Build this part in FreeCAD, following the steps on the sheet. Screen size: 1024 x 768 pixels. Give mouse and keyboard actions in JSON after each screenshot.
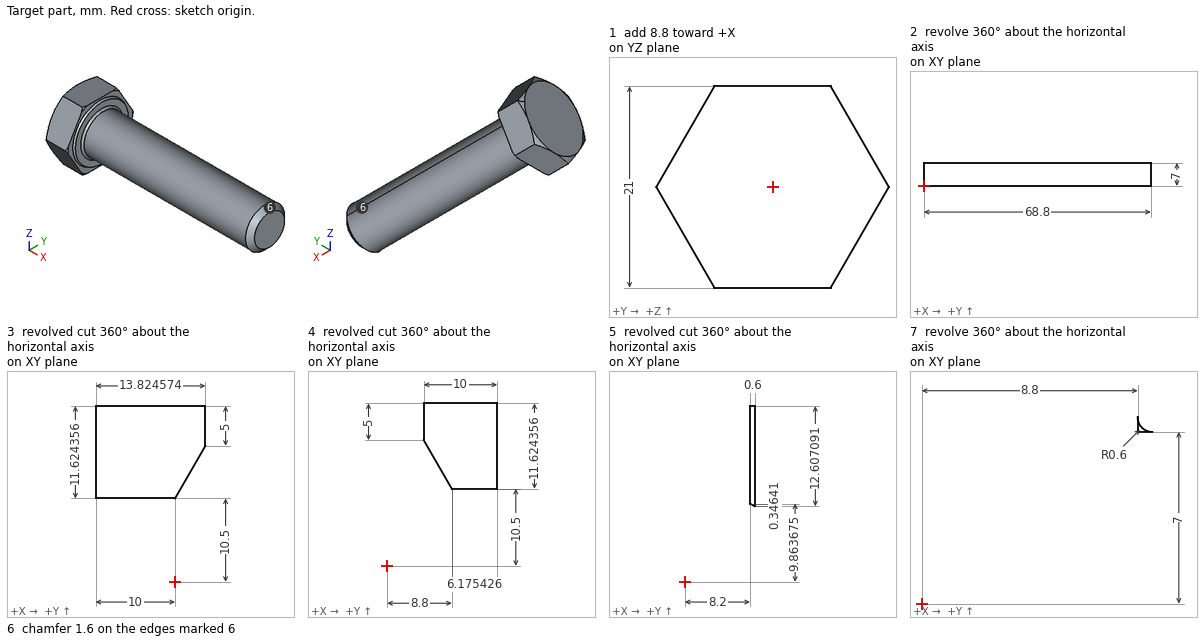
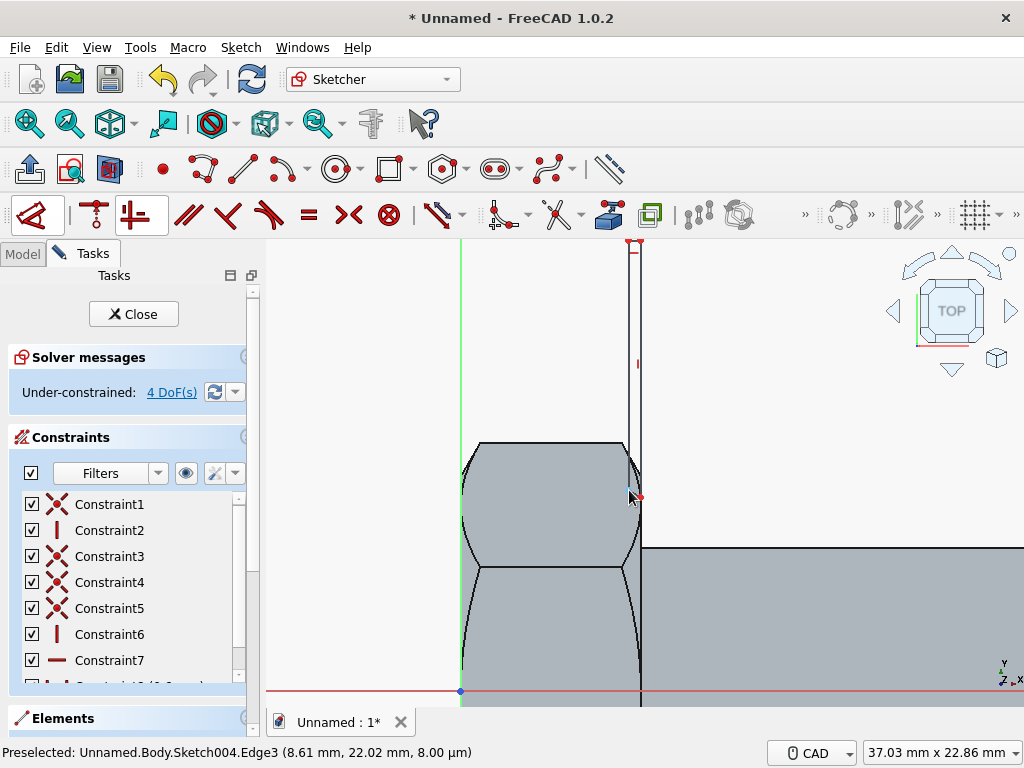
{"action": "left_click", "coordinate": [629, 490]}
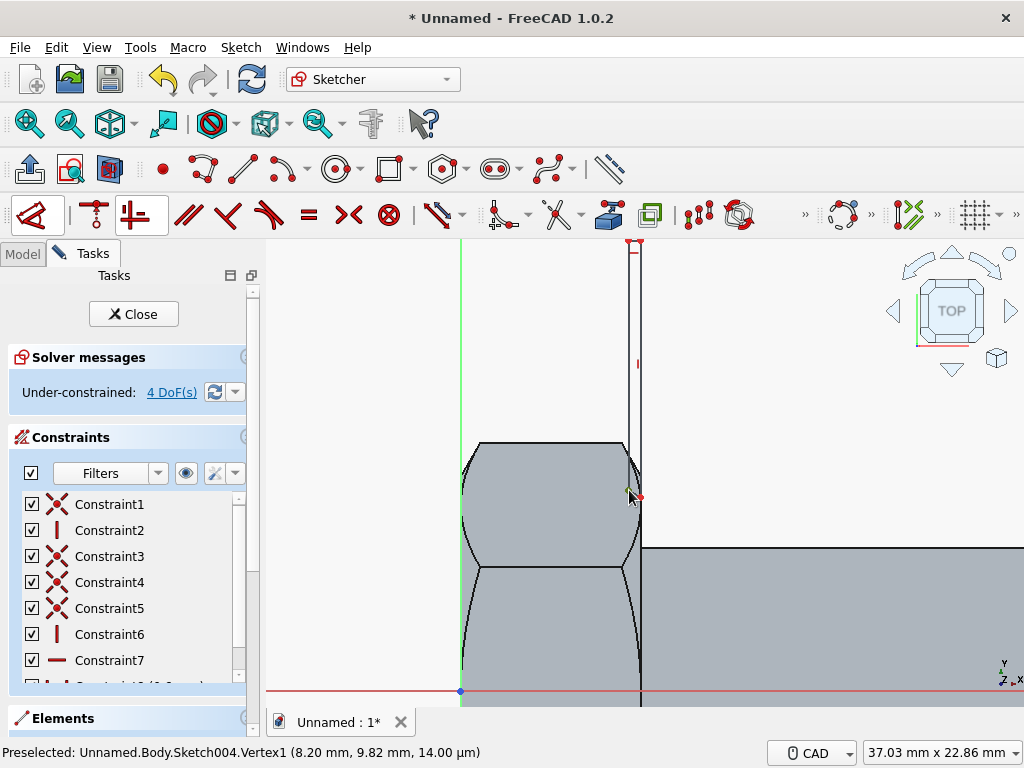
{"action": "left_click", "coordinate": [58, 216]}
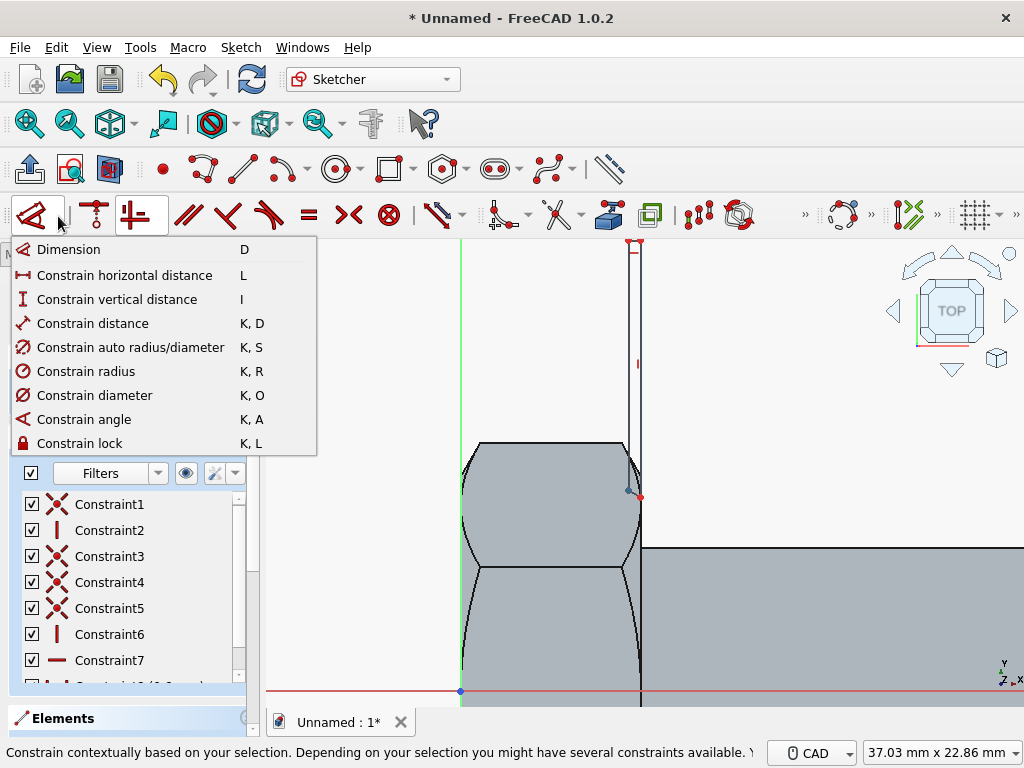
{"action": "left_click", "coordinate": [164, 275]}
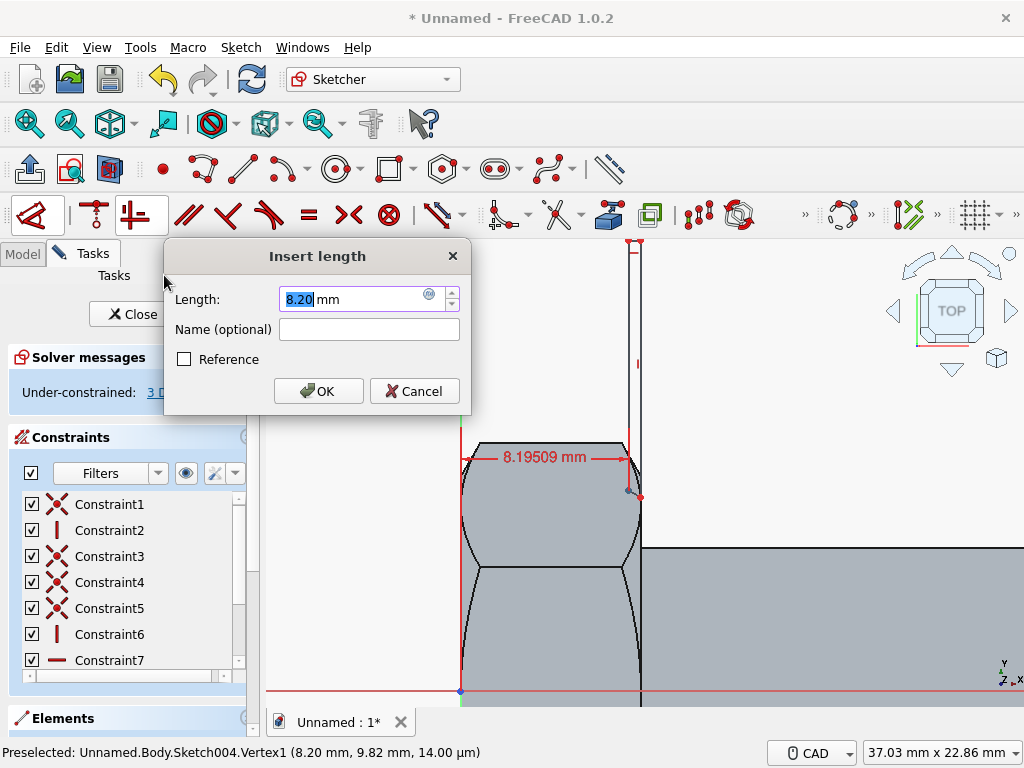
{"action": "type", "text": "8.2"}
{"action": "key", "text": "Return"}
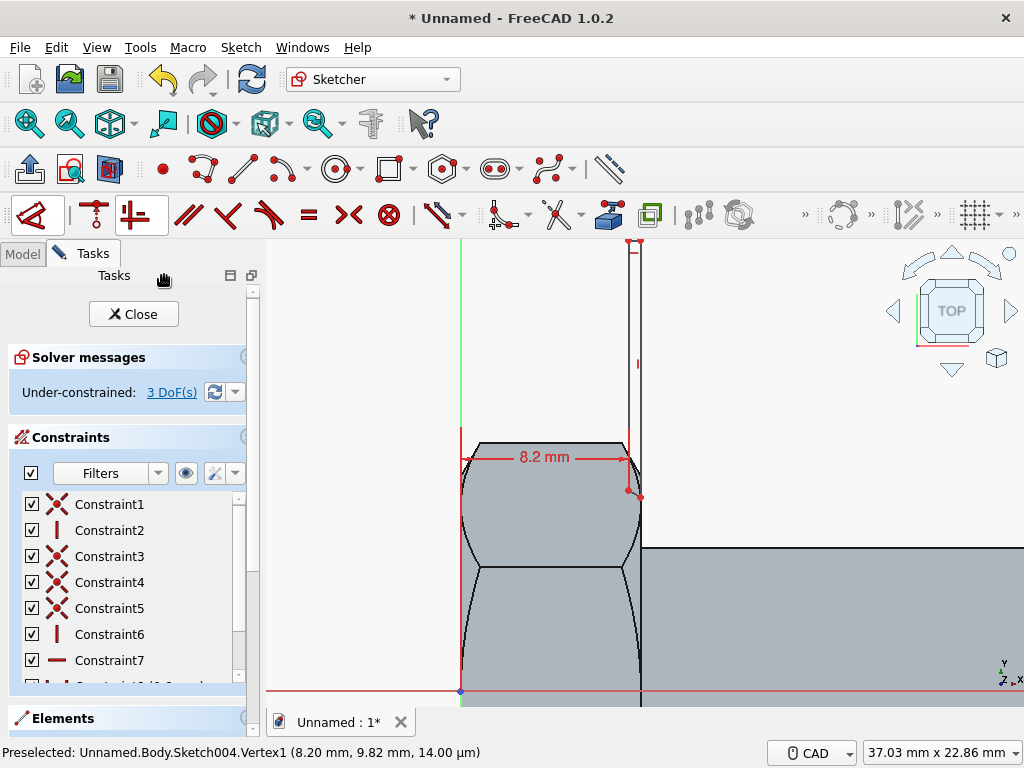
{"action": "scroll", "coordinate": [635, 494], "scroll_direction": "up", "scroll_amount": 9}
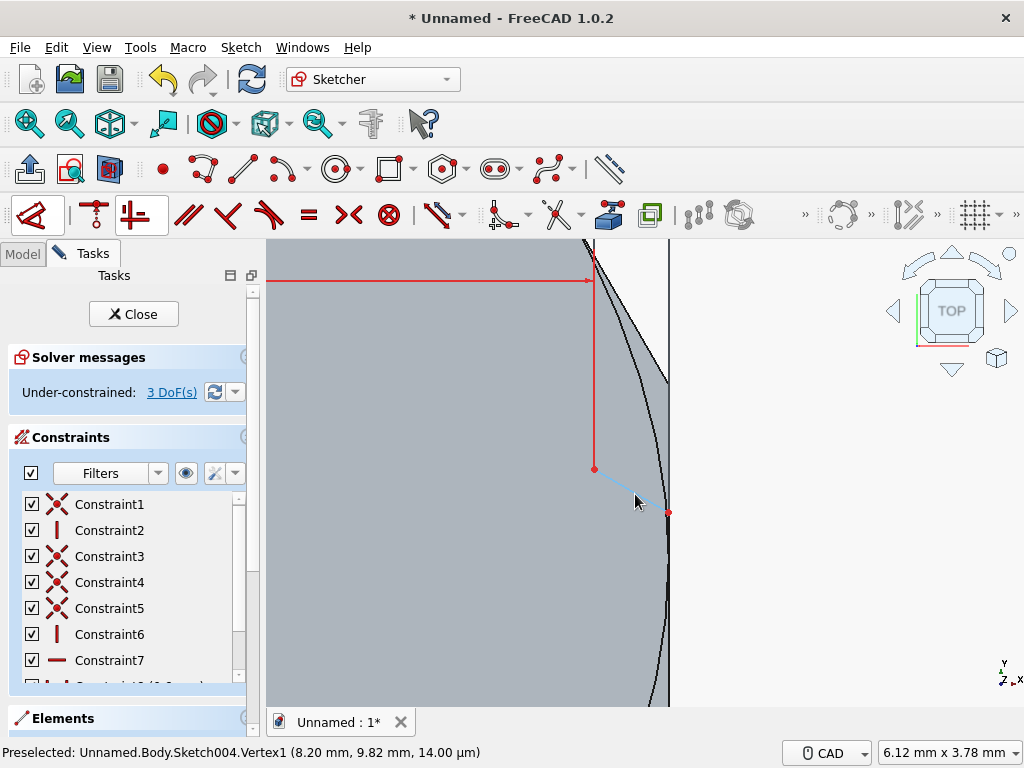
{"action": "left_click", "coordinate": [632, 491]}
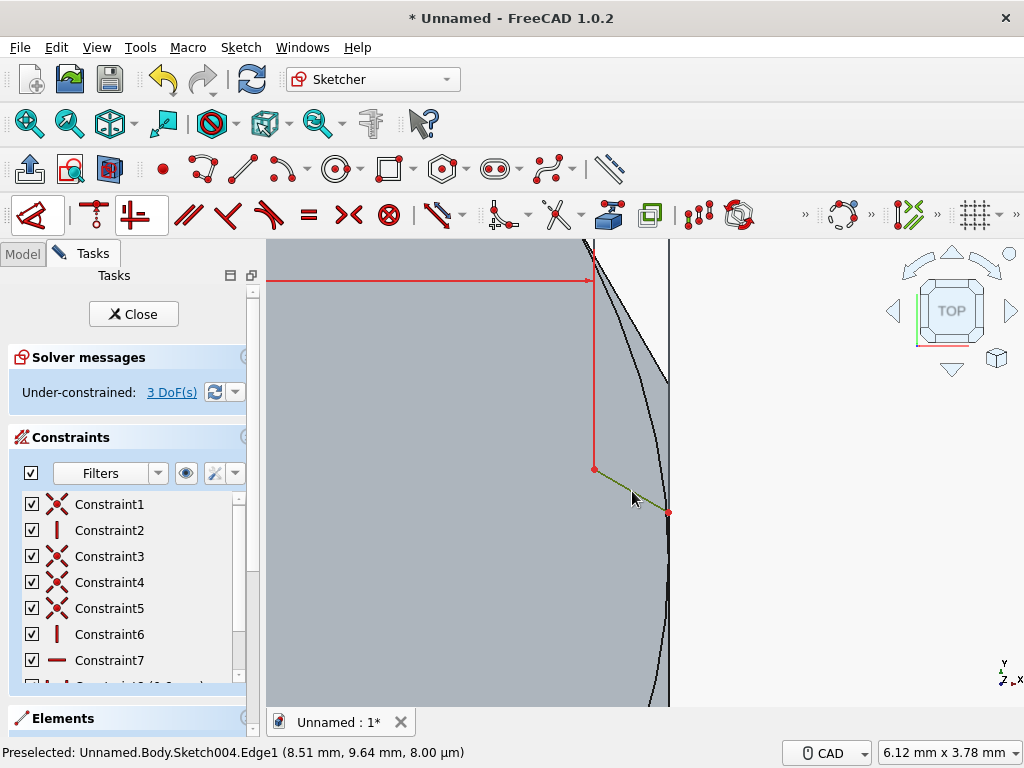
{"action": "key", "text": "i"}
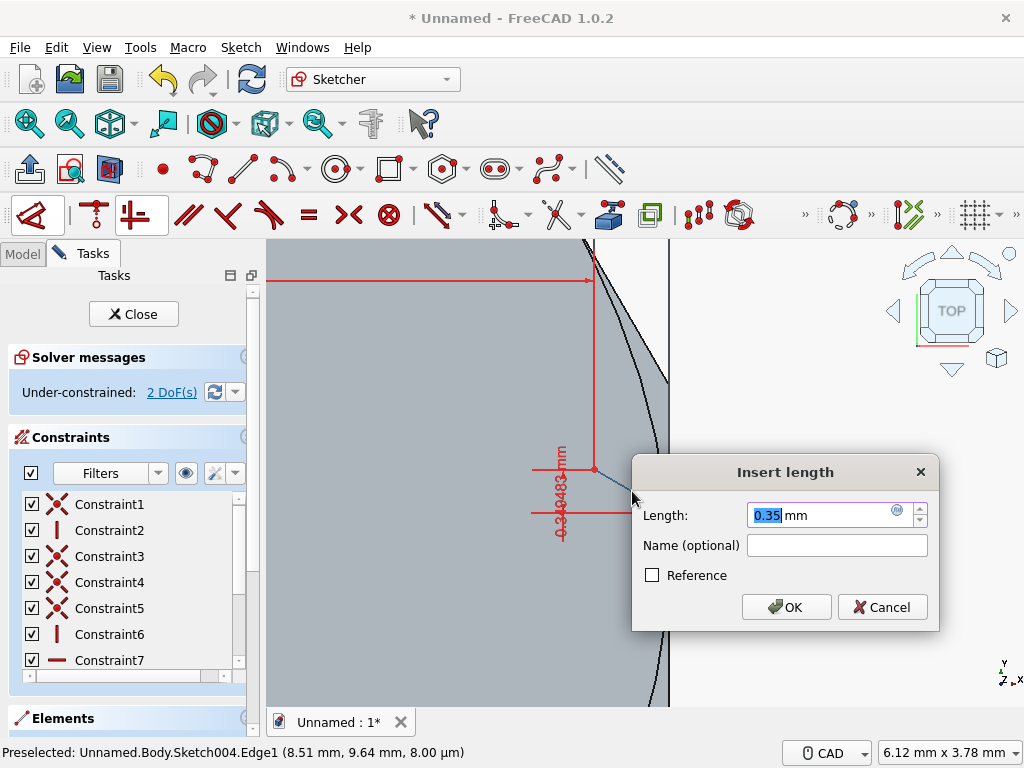
{"action": "type", "text": "0.34641"}
{"action": "key", "text": "Return"}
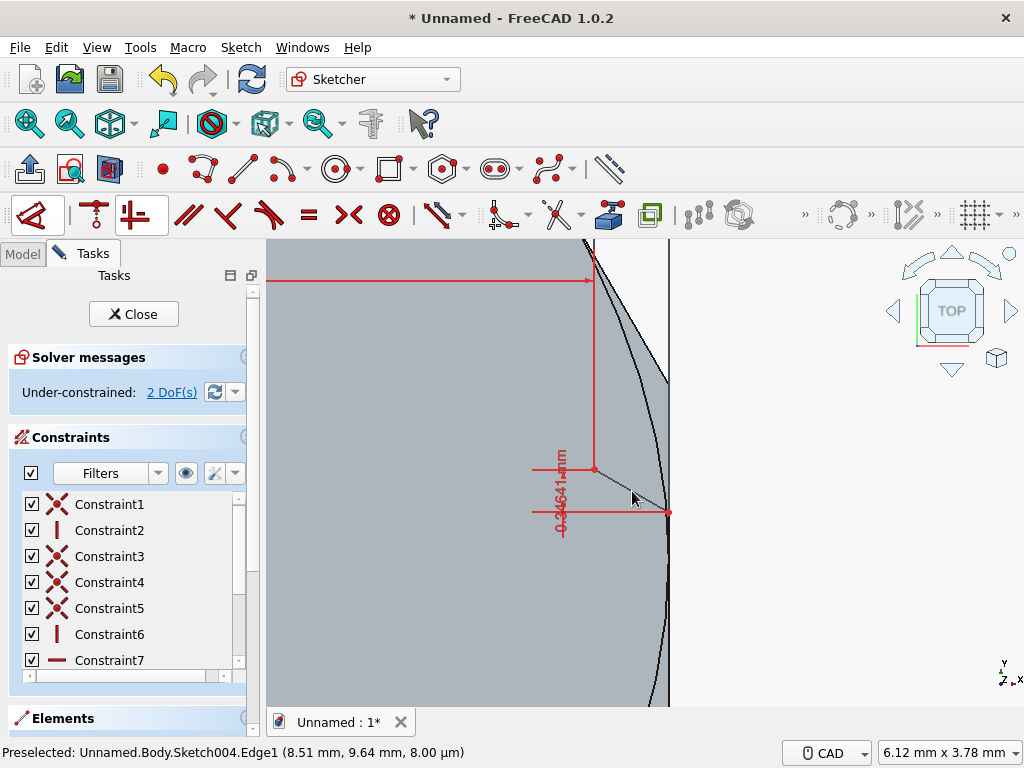
{"action": "scroll", "coordinate": [633, 493], "scroll_direction": "down", "scroll_amount": 11}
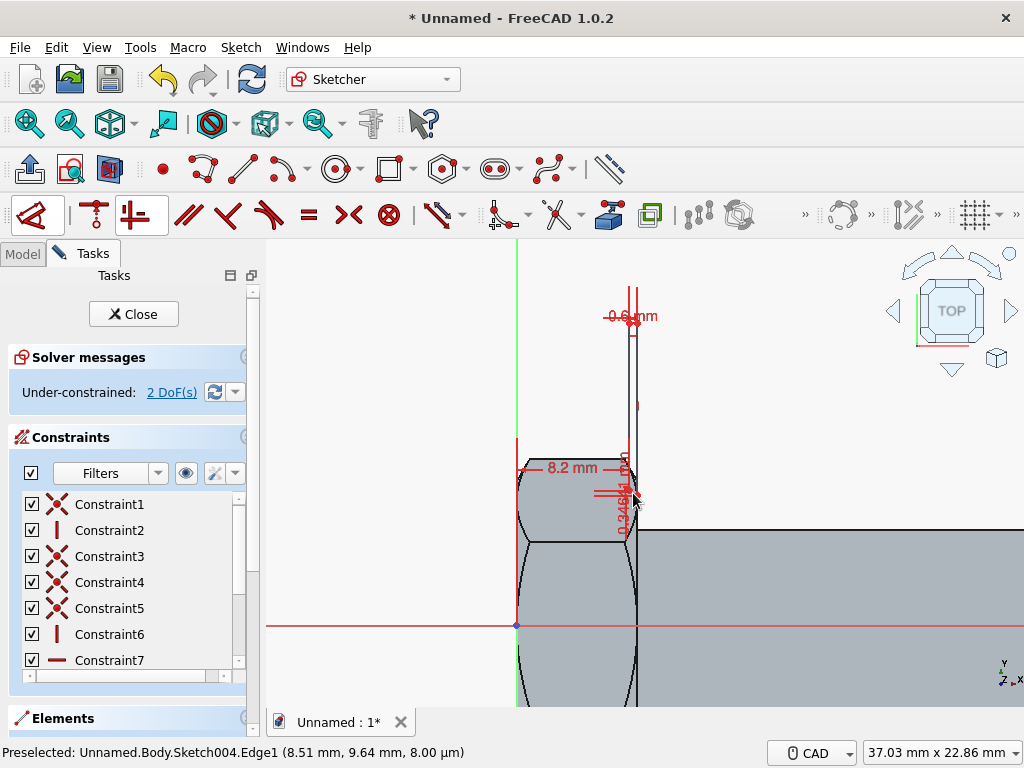
{"action": "scroll", "coordinate": [637, 444], "scroll_direction": "up", "scroll_amount": 3}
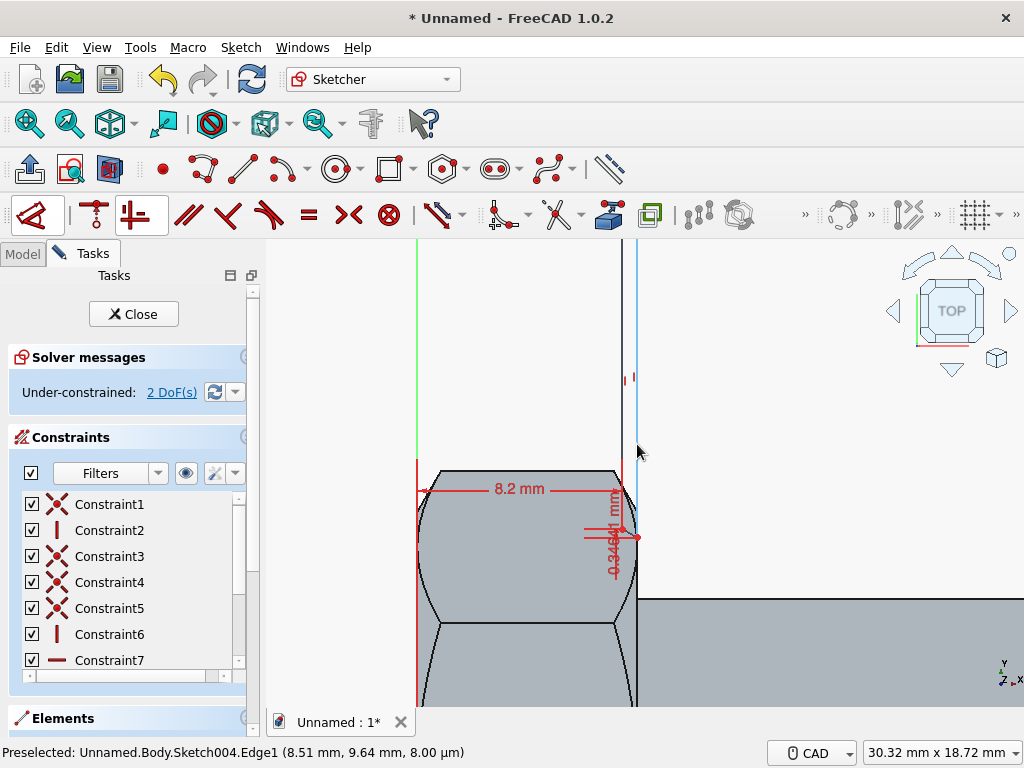
{"action": "left_click", "coordinate": [637, 444]}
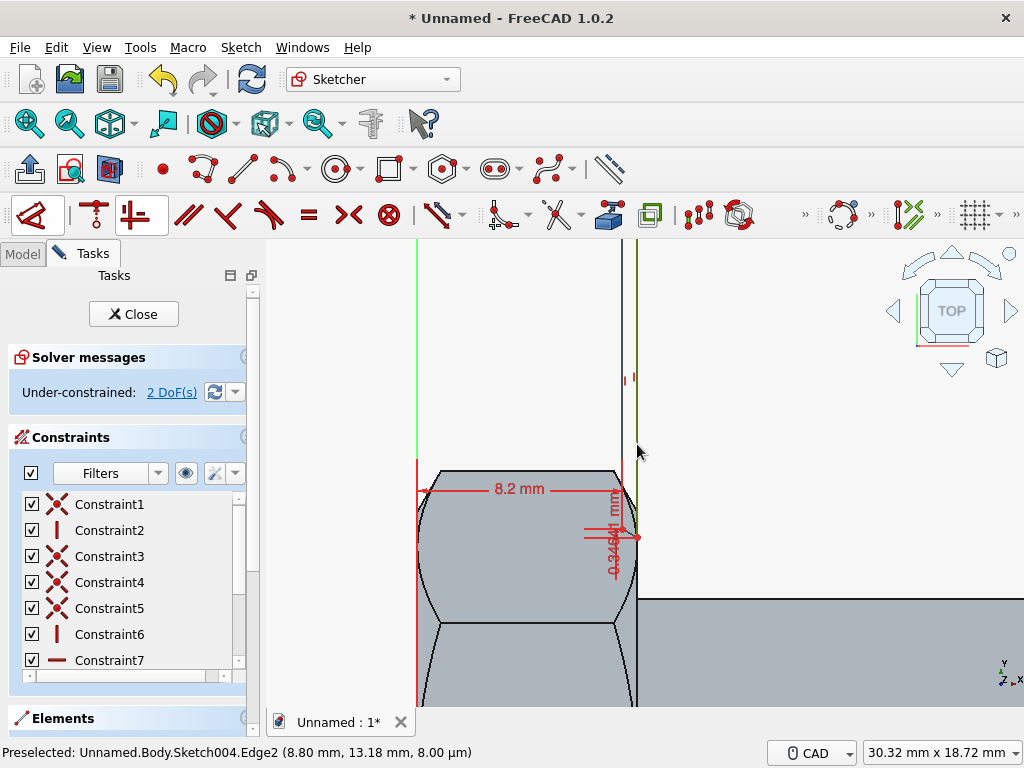
{"action": "key", "text": "i"}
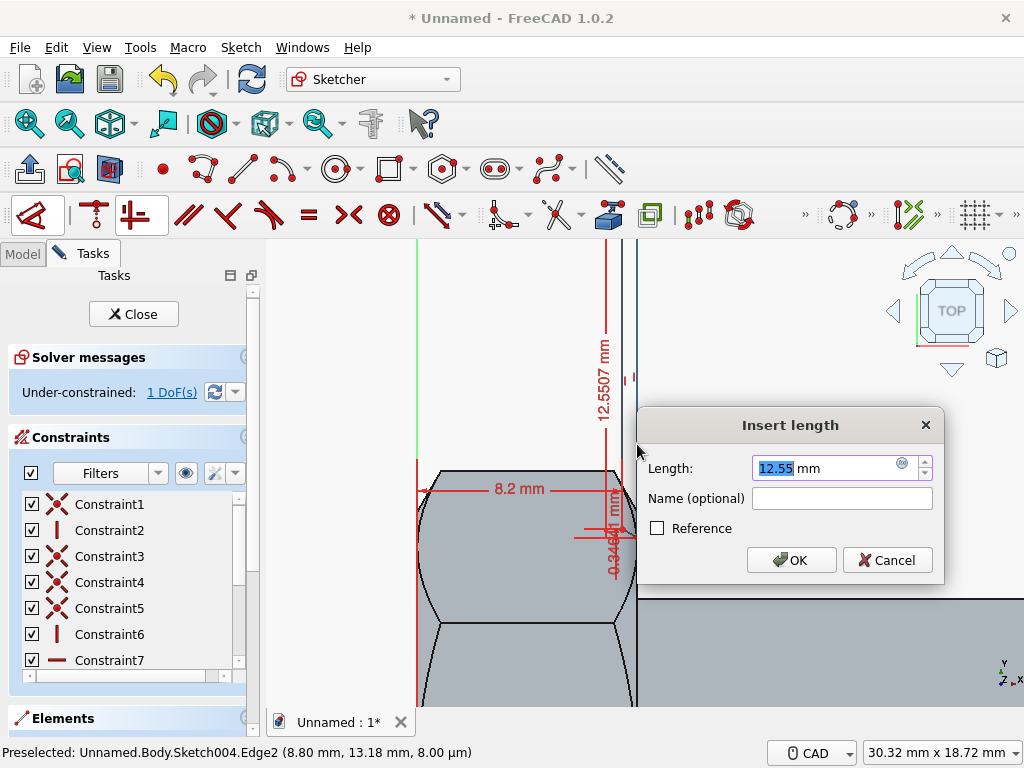
{"action": "type", "text": "12.607091"}
{"action": "key", "text": "Return"}